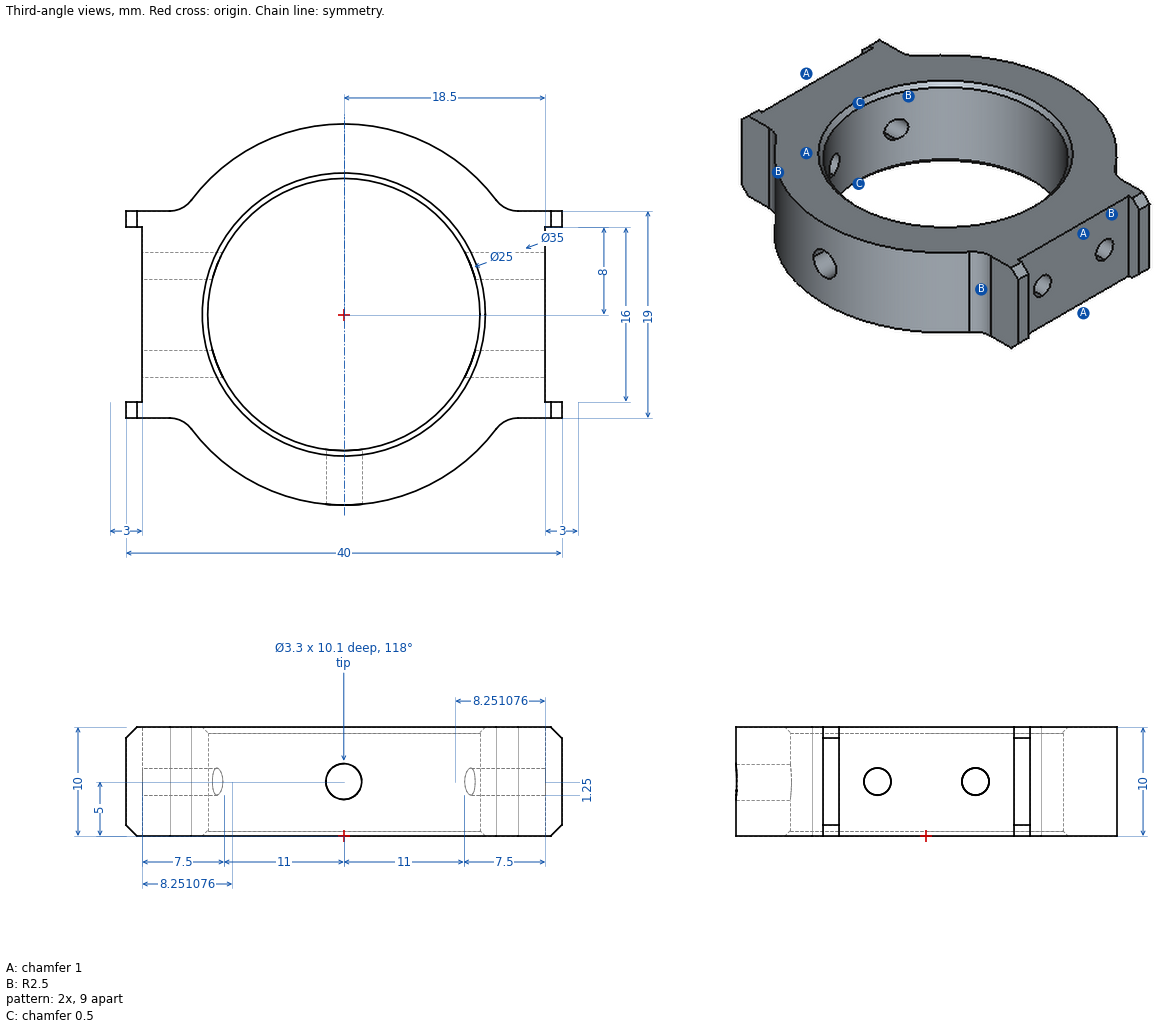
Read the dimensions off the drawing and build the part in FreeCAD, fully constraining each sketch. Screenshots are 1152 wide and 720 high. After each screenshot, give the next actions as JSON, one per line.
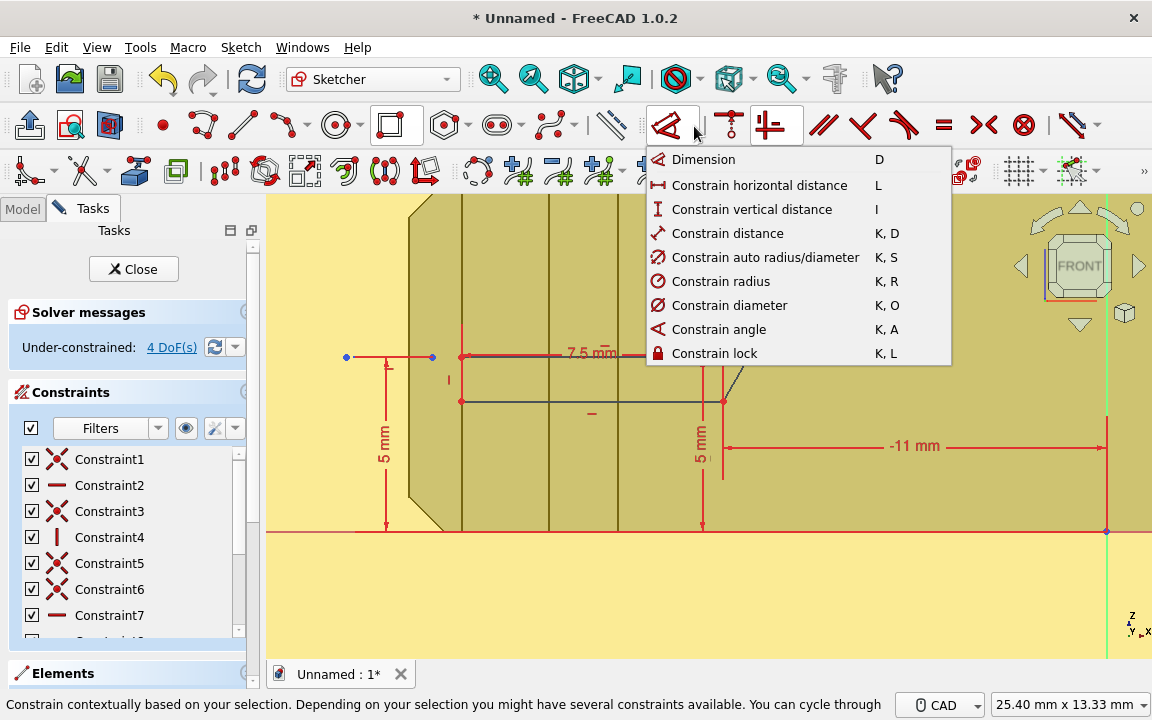
{"action": "left_click", "coordinate": [799, 209]}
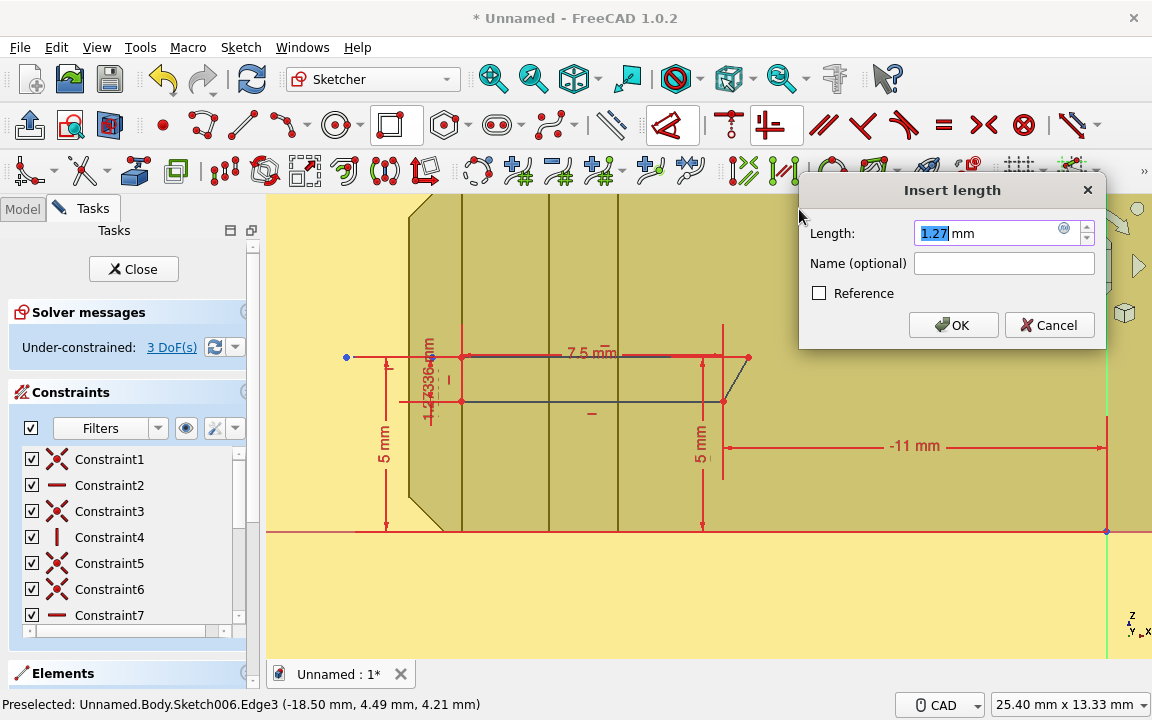
{"action": "type", "text": "1.25"}
{"action": "key", "text": "Return"}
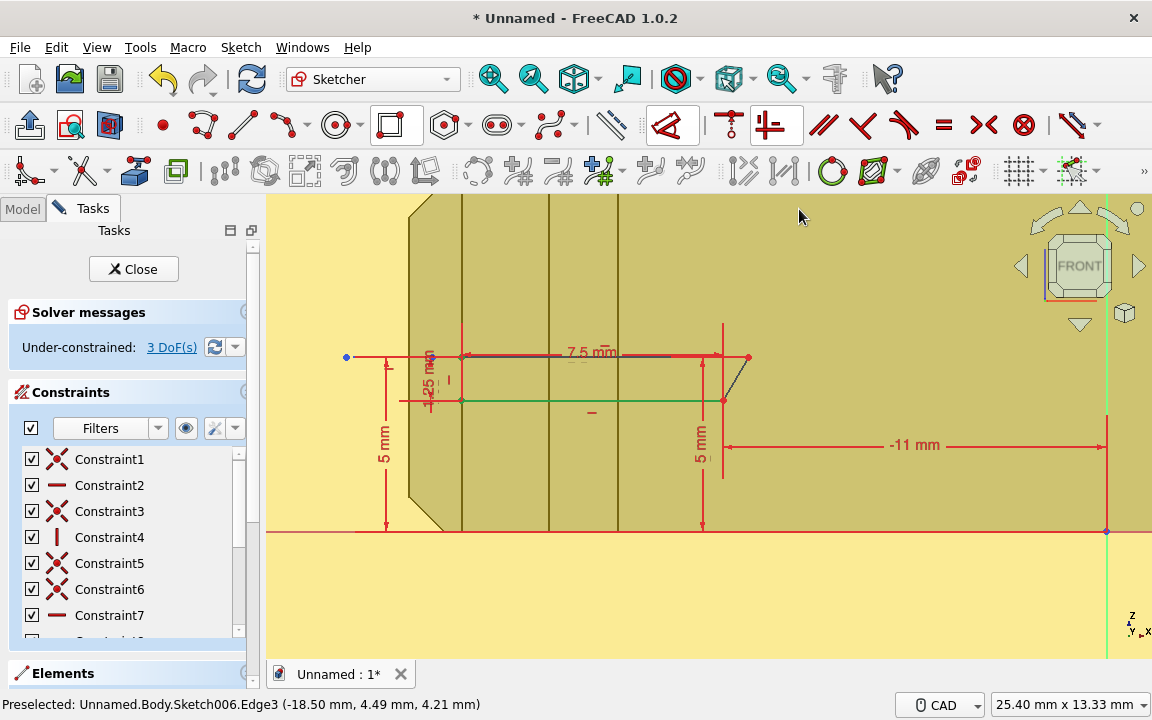
{"action": "left_click", "coordinate": [548, 357]}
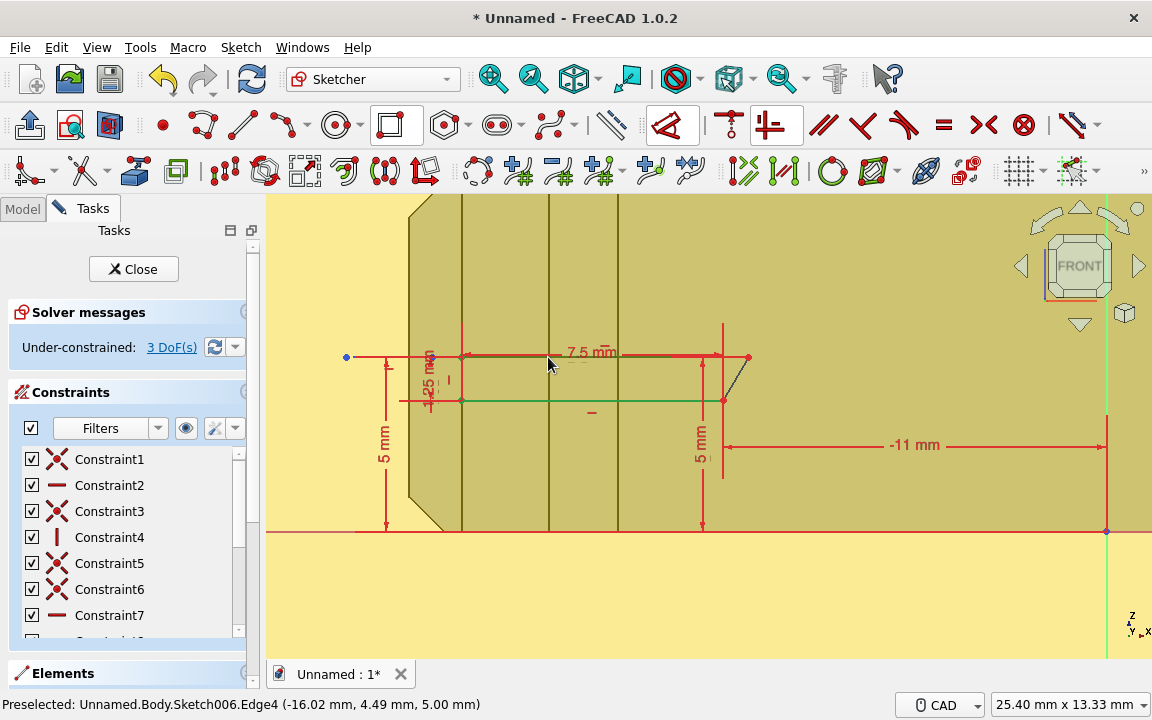
{"action": "left_click", "coordinate": [694, 126]}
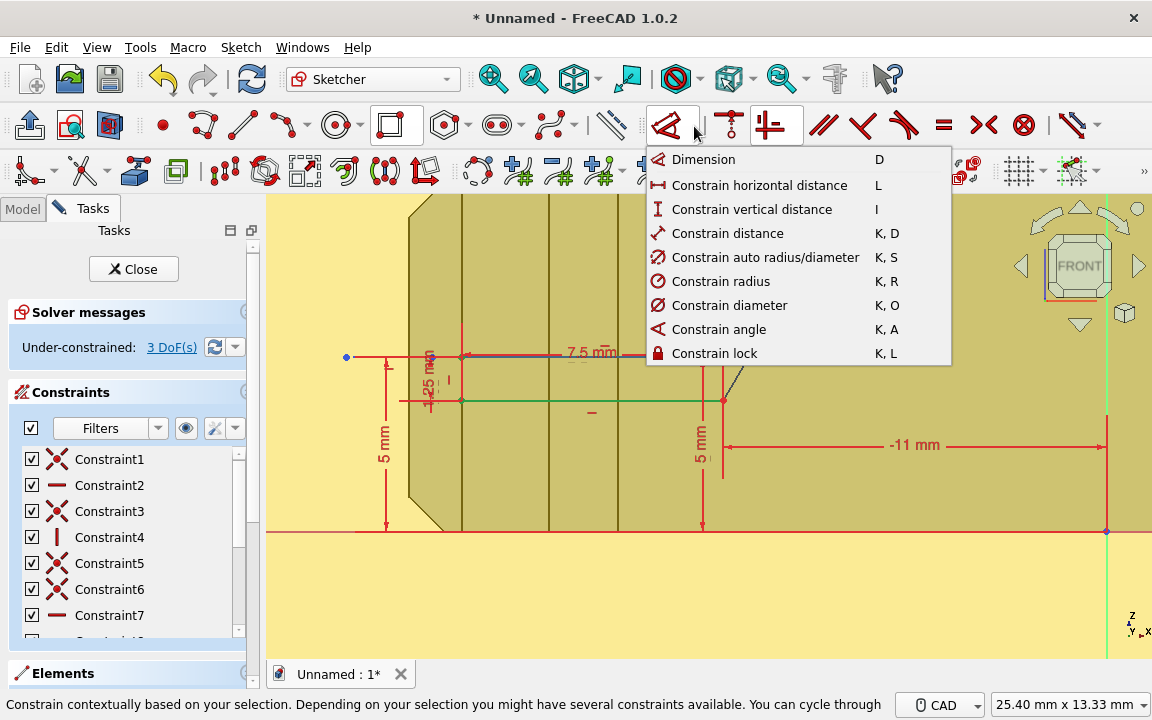
{"action": "left_click", "coordinate": [799, 185]}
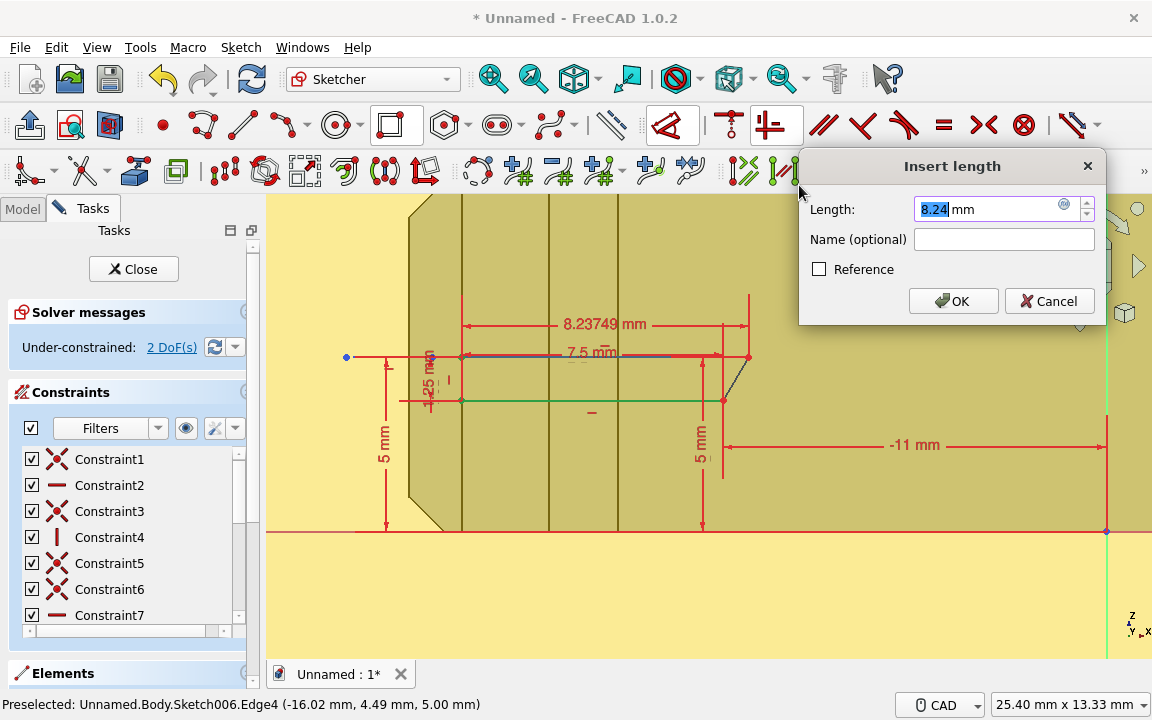
{"action": "type", "text": "8.251076"}
{"action": "key", "text": "Return"}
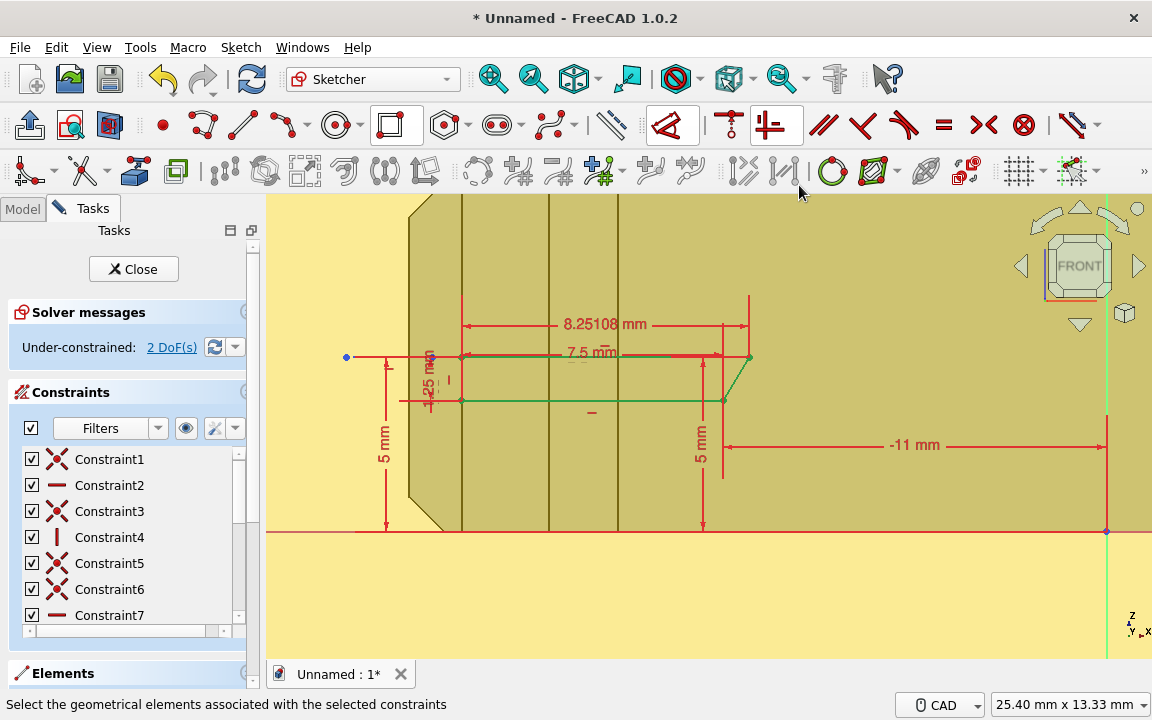
{"action": "left_click", "coordinate": [134, 269]}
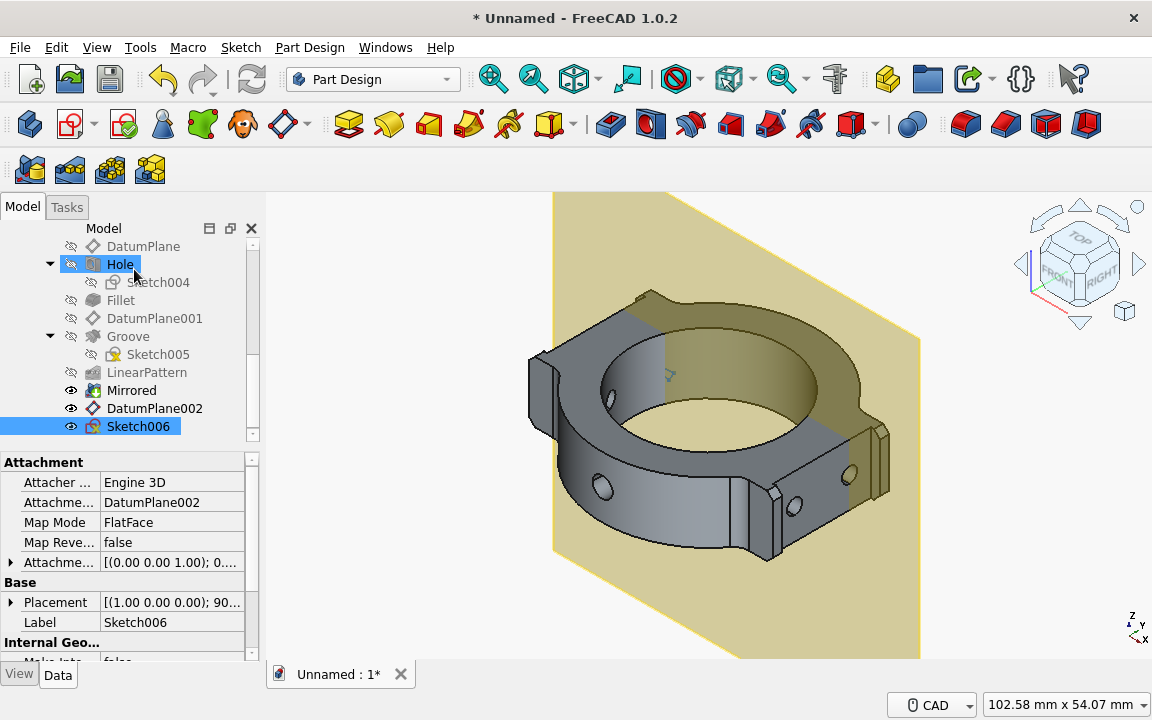
{"action": "left_click", "coordinate": [692, 124]}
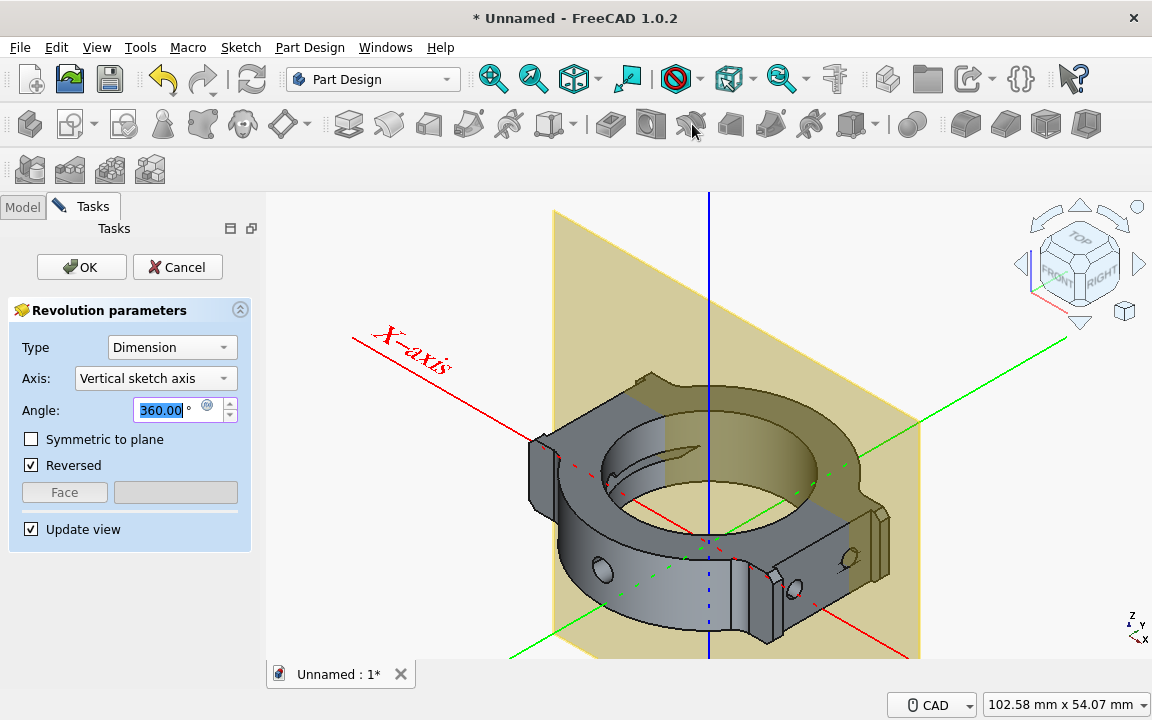
{"action": "left_click", "coordinate": [156, 378]}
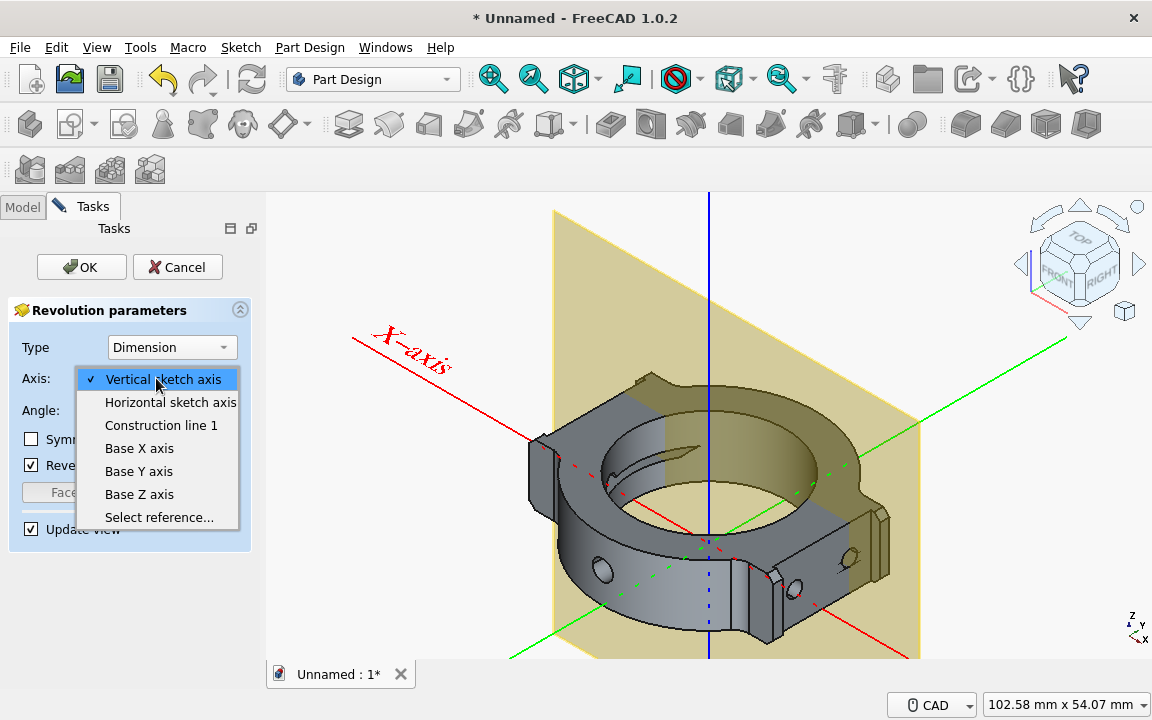
{"action": "left_click", "coordinate": [156, 426]}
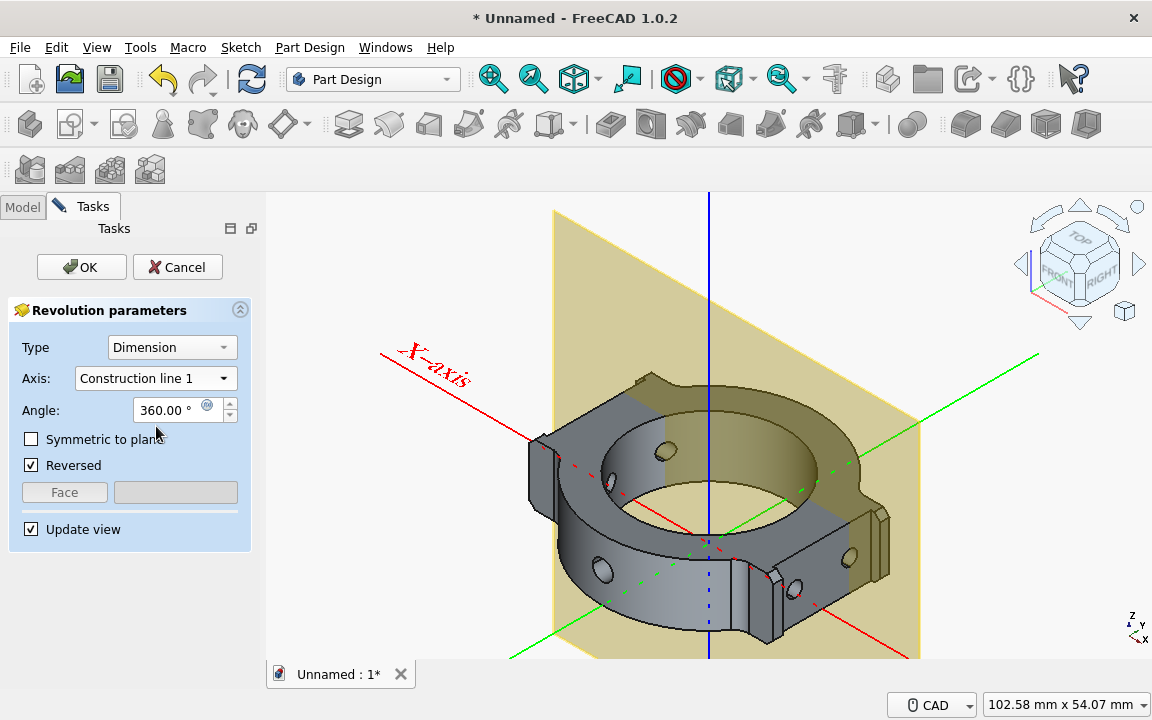
{"action": "left_click", "coordinate": [82, 267]}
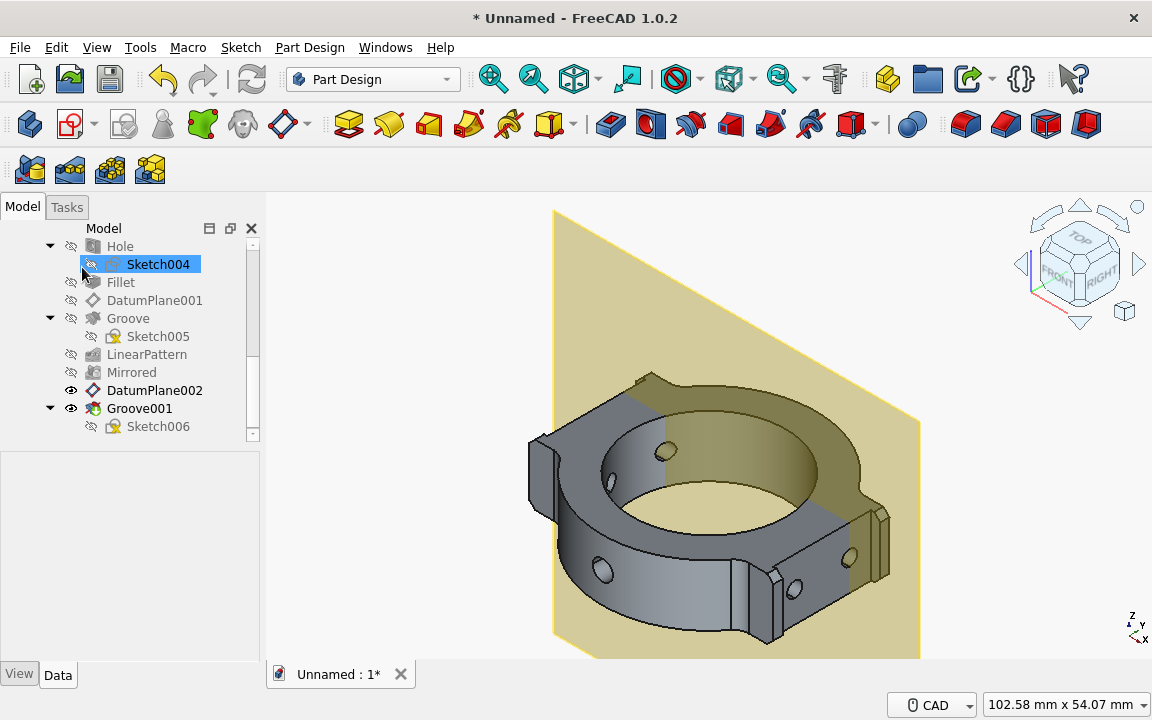
{"action": "left_click", "coordinate": [116, 390]}
{"action": "key", "text": "space"}